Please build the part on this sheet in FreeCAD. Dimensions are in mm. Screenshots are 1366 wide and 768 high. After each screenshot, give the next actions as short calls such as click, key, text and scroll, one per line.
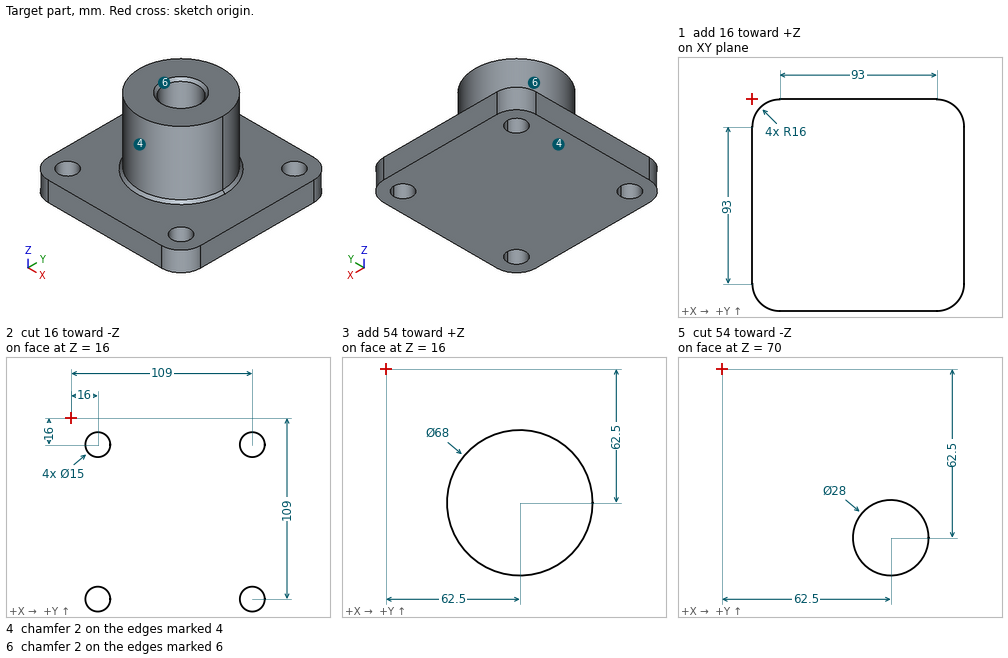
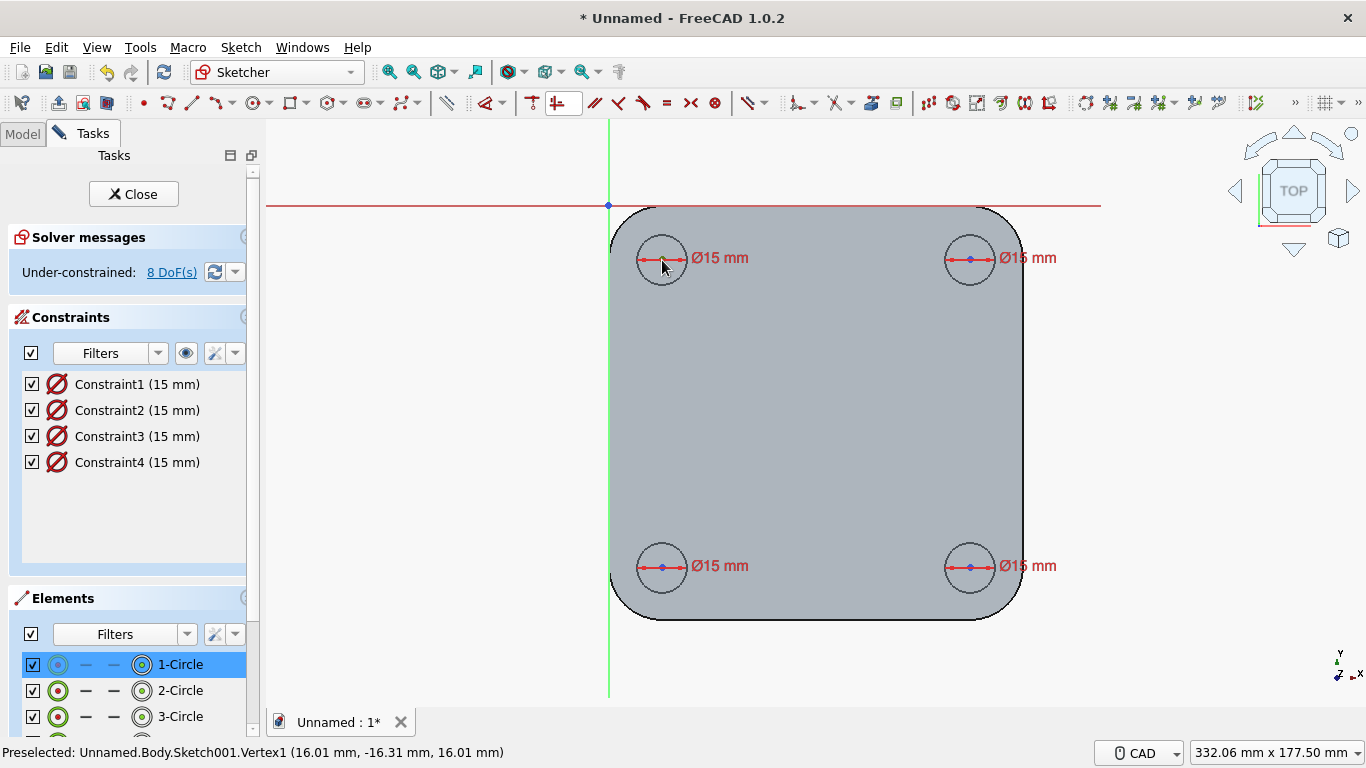
click(970, 260)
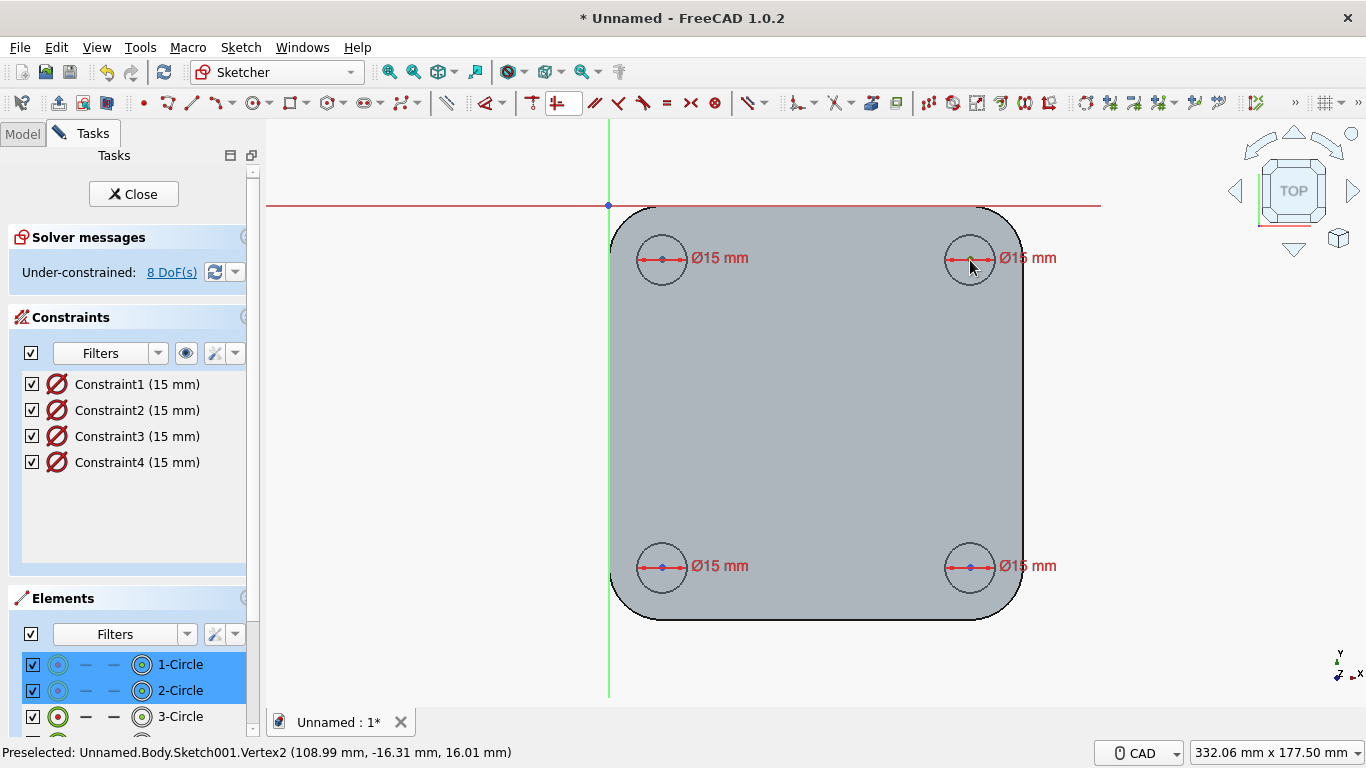
key(h)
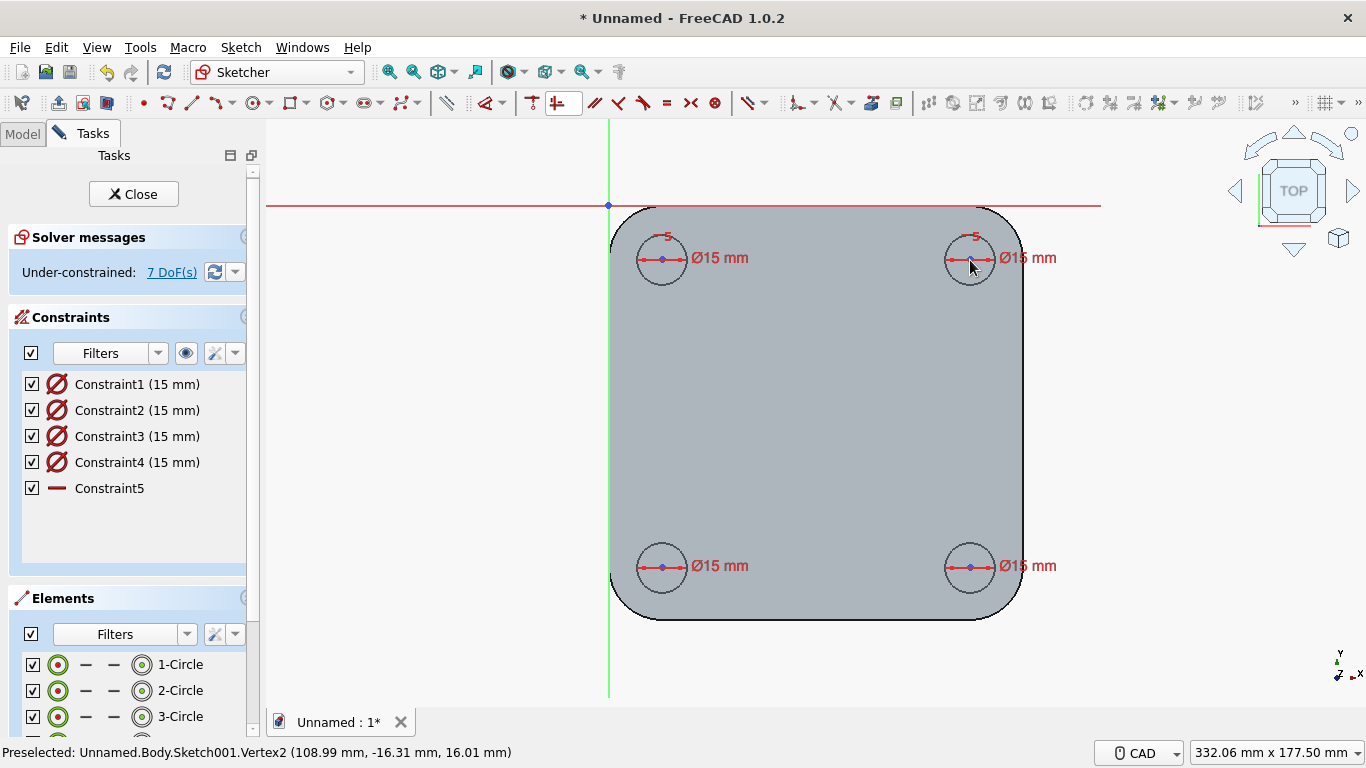
click(970, 260)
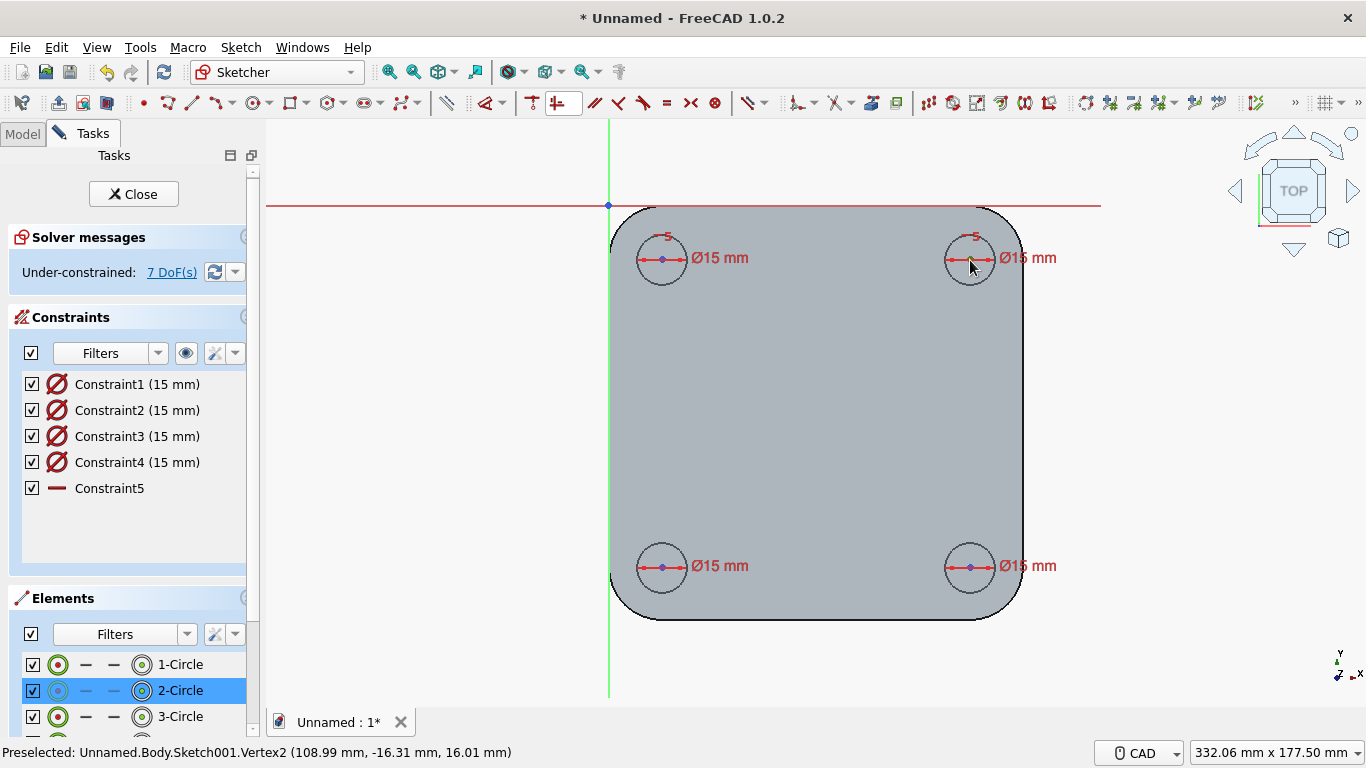
click(970, 568)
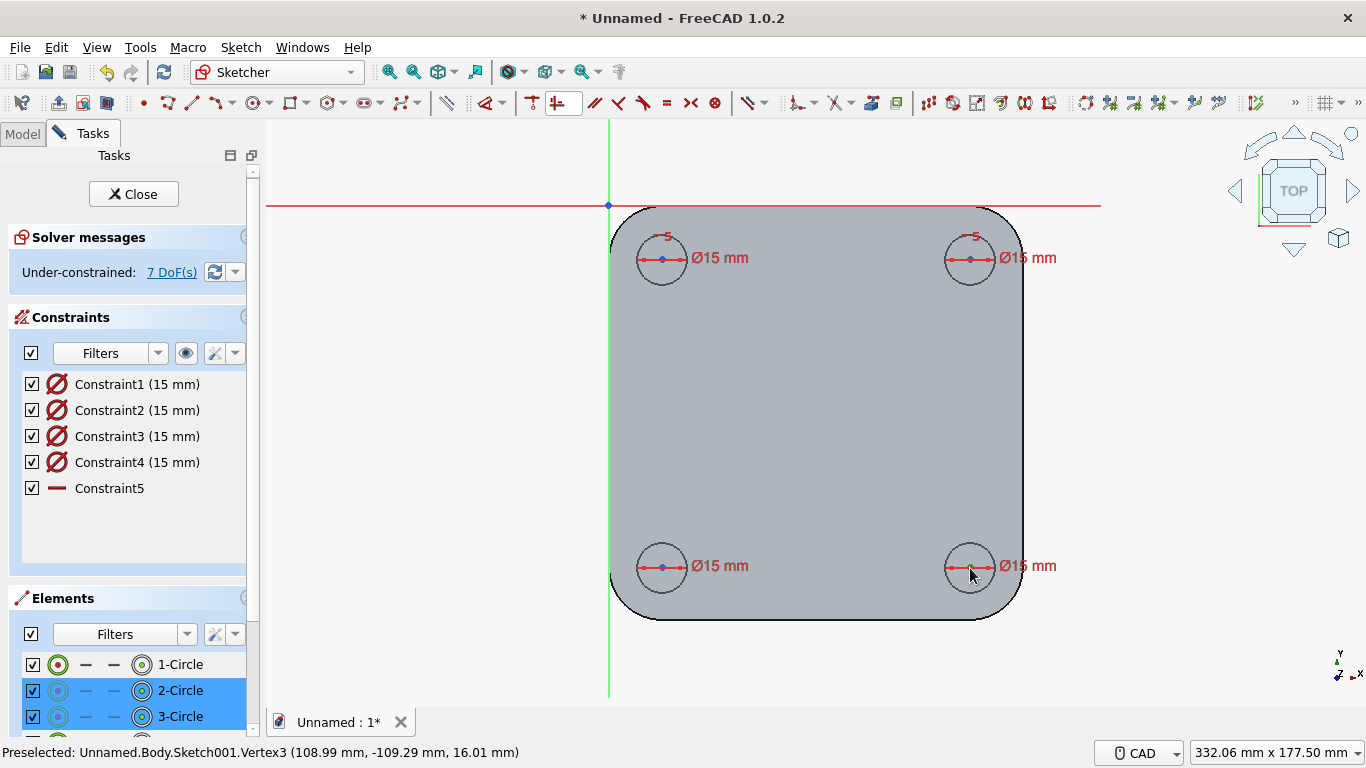
click(576, 104)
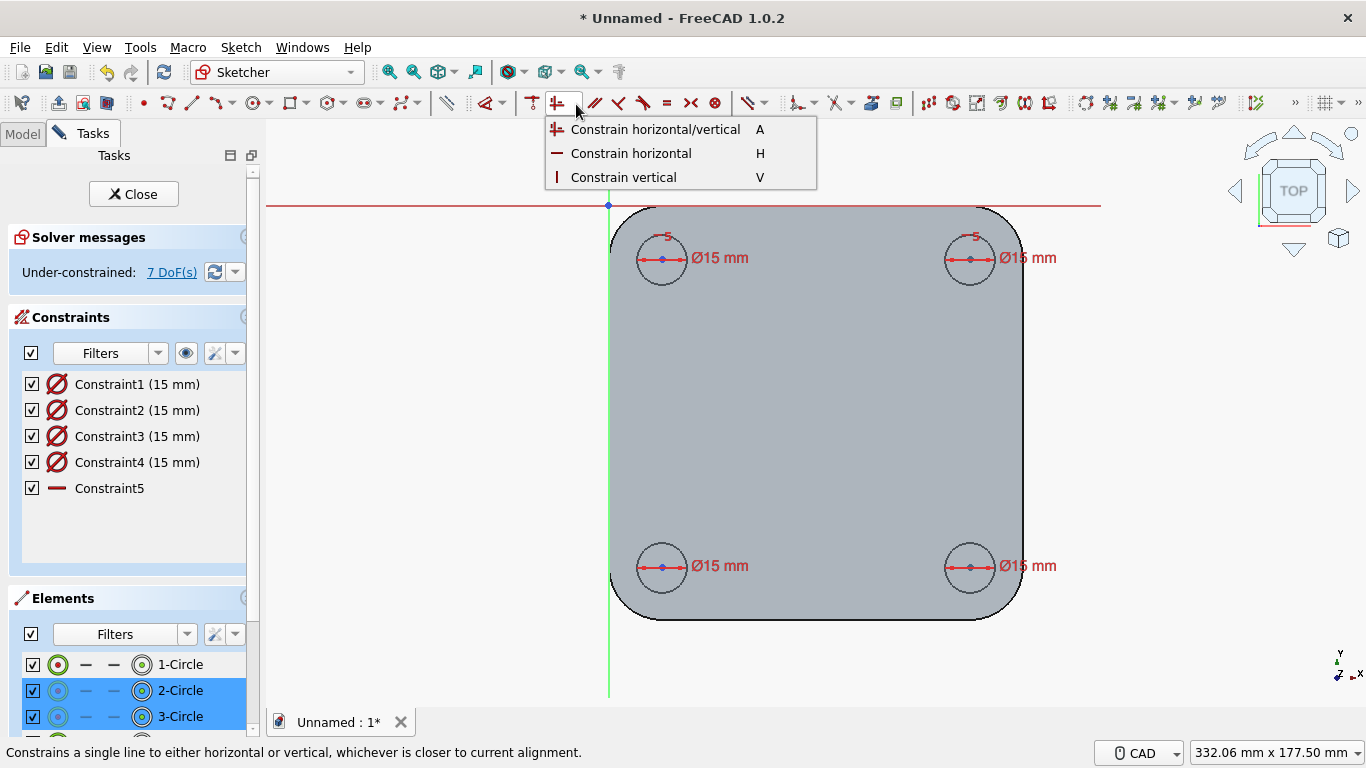
click(681, 177)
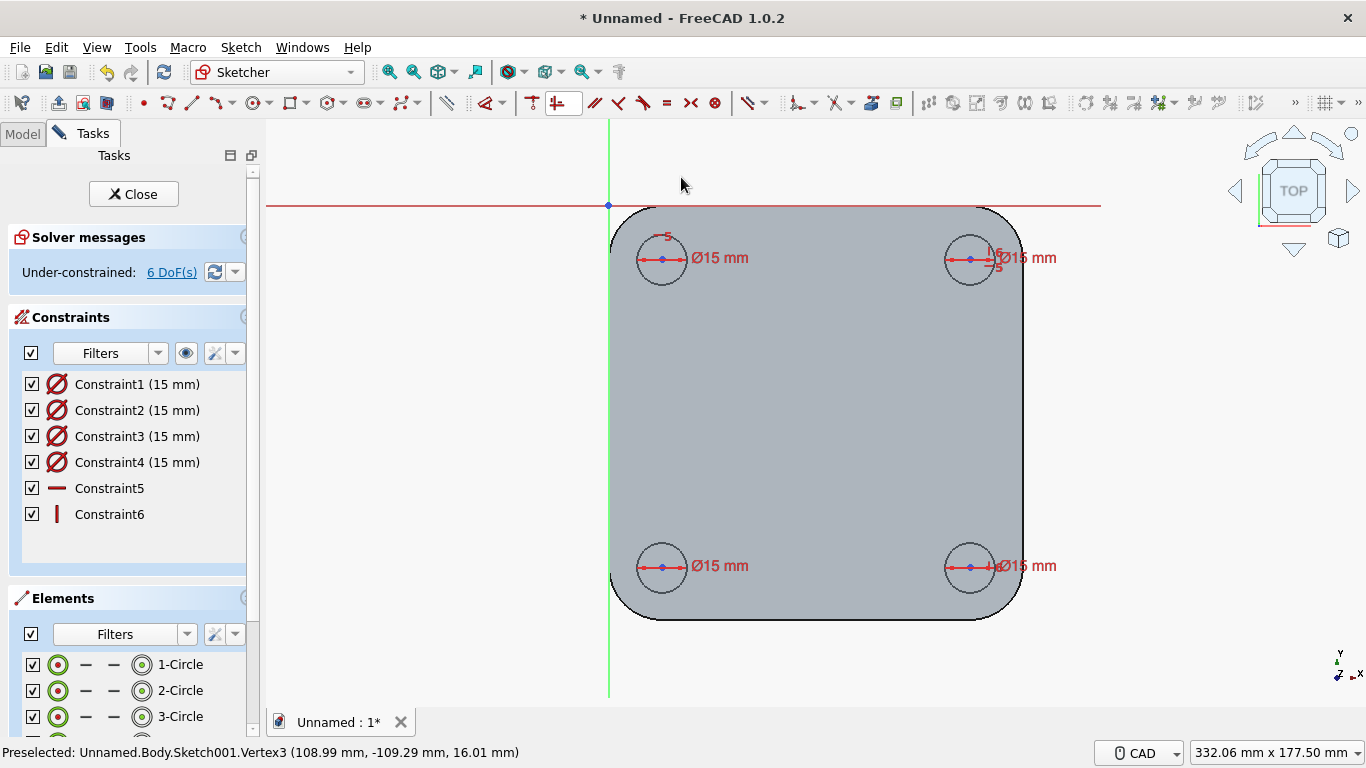
click(662, 260)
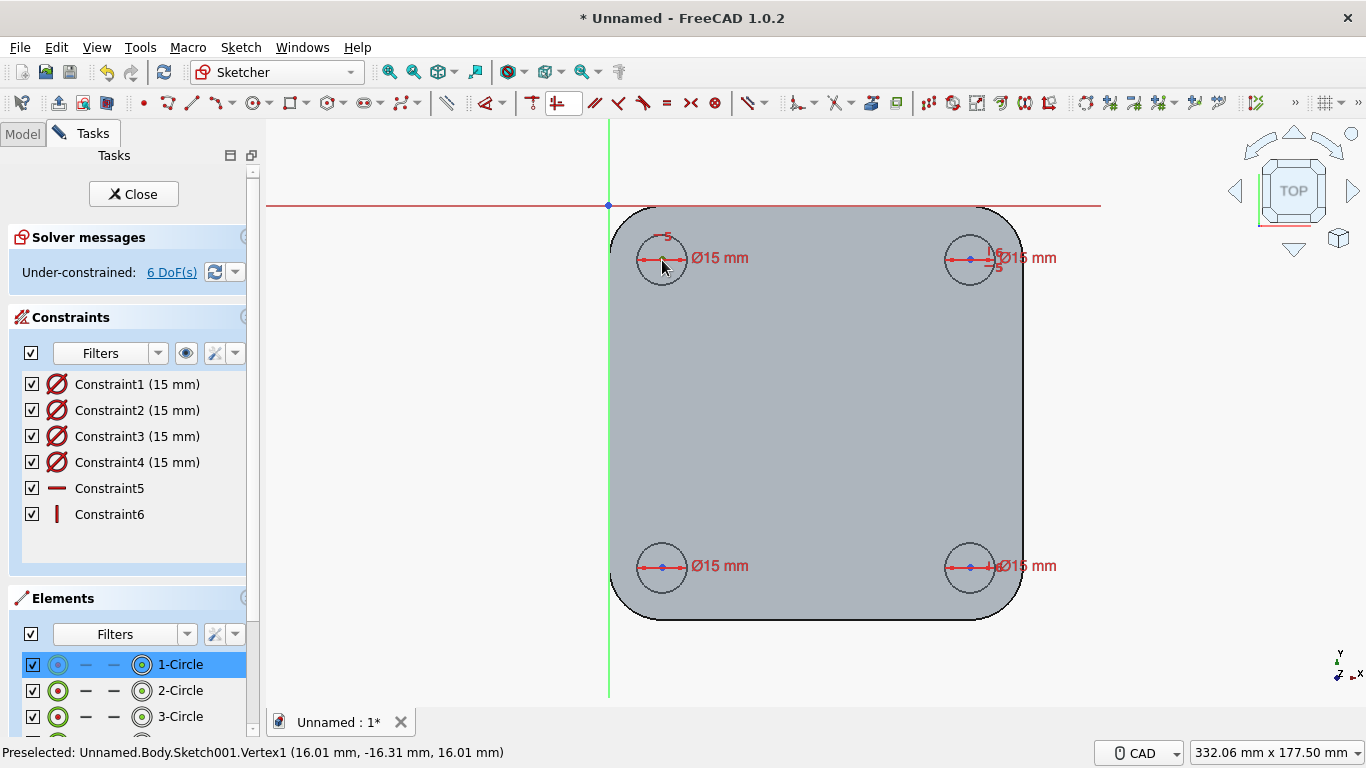
click(662, 568)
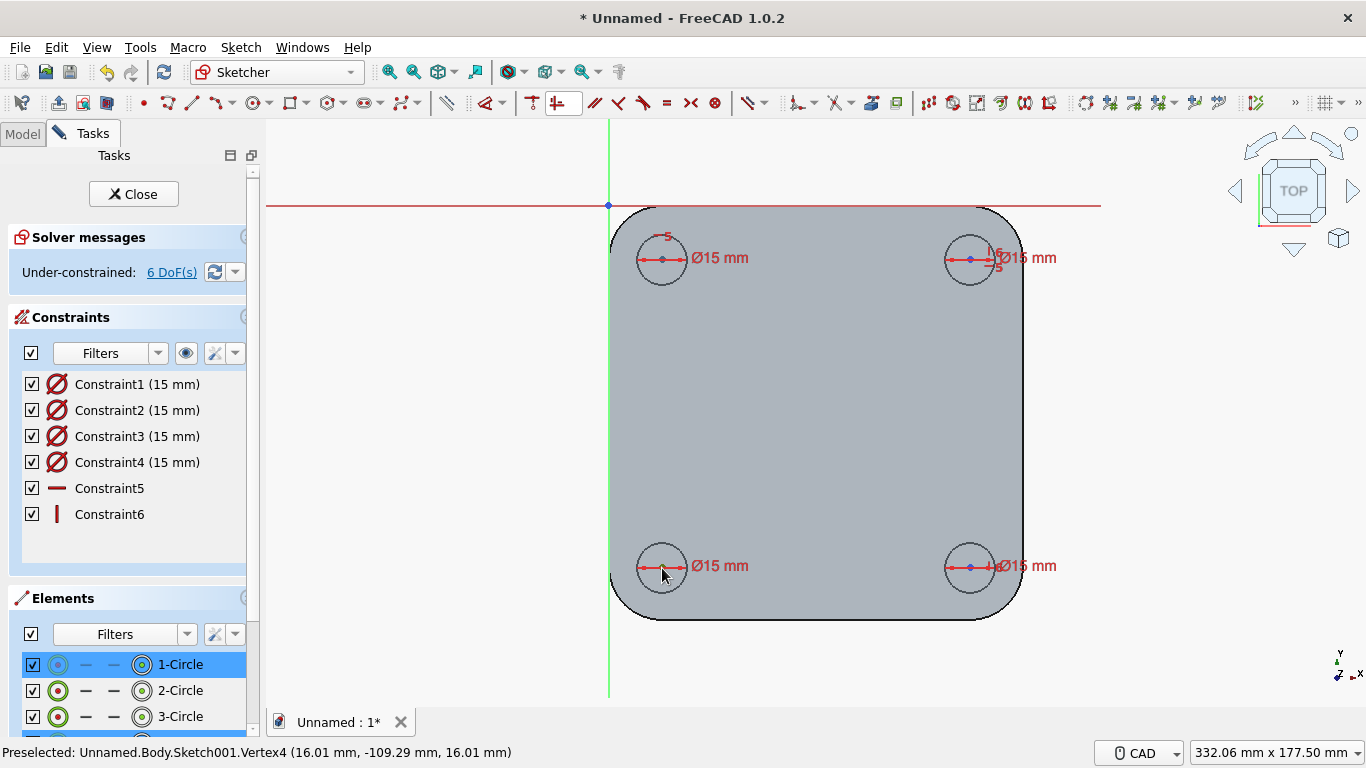
click(576, 104)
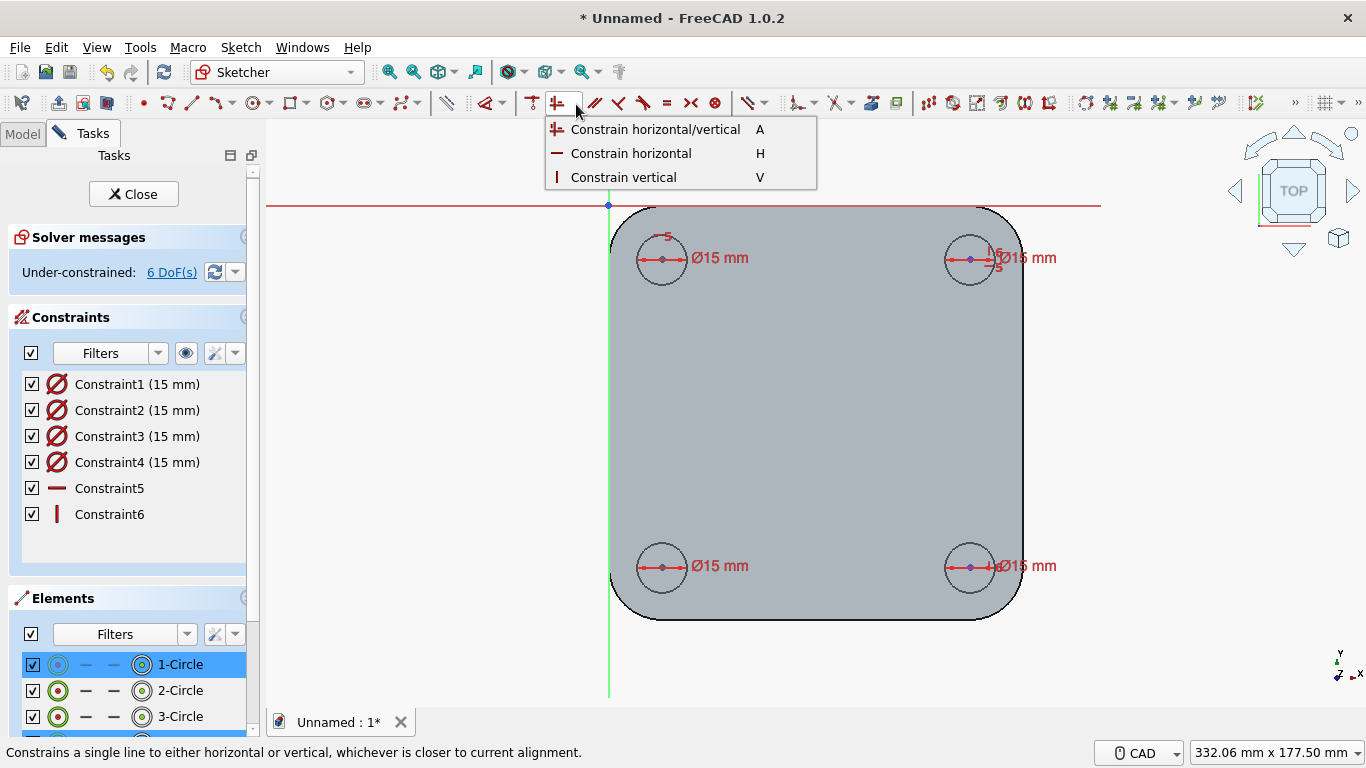
click(681, 177)